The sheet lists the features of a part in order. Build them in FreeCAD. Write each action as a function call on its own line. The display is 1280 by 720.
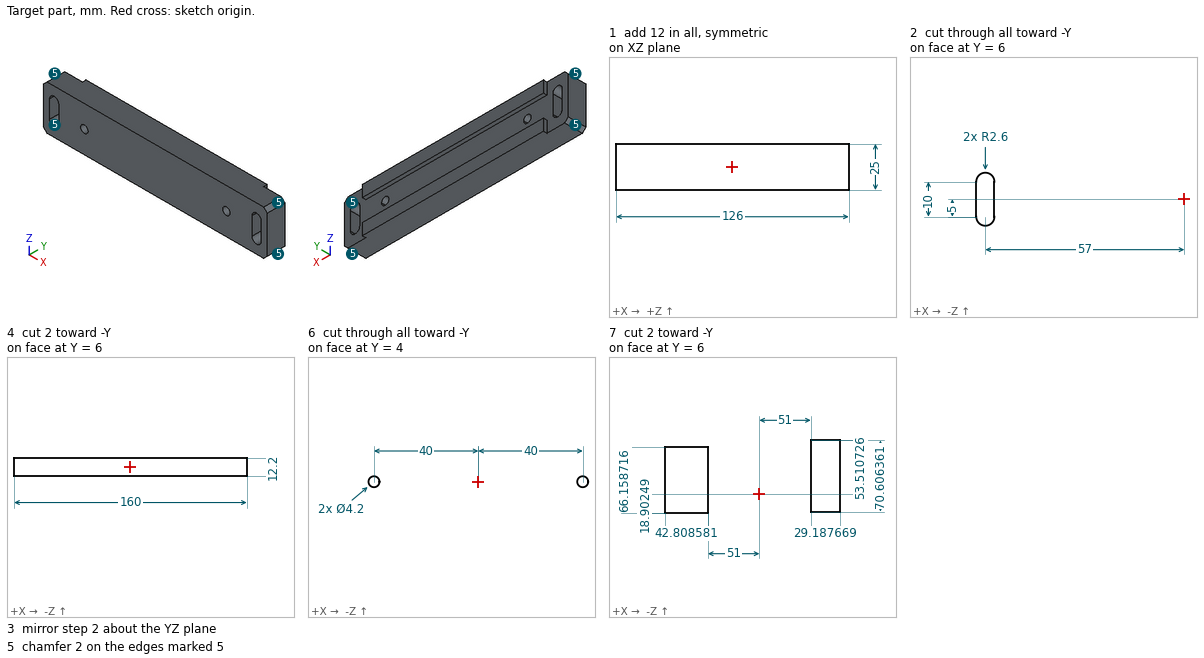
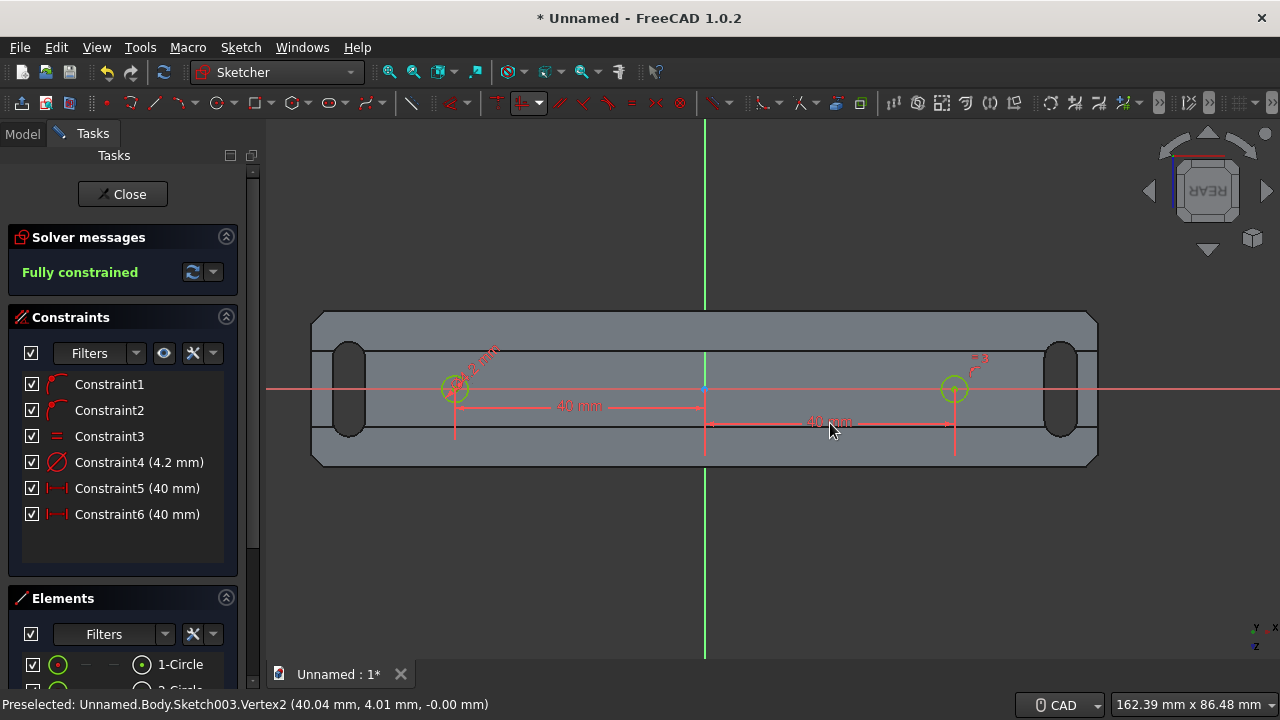
click(123, 194)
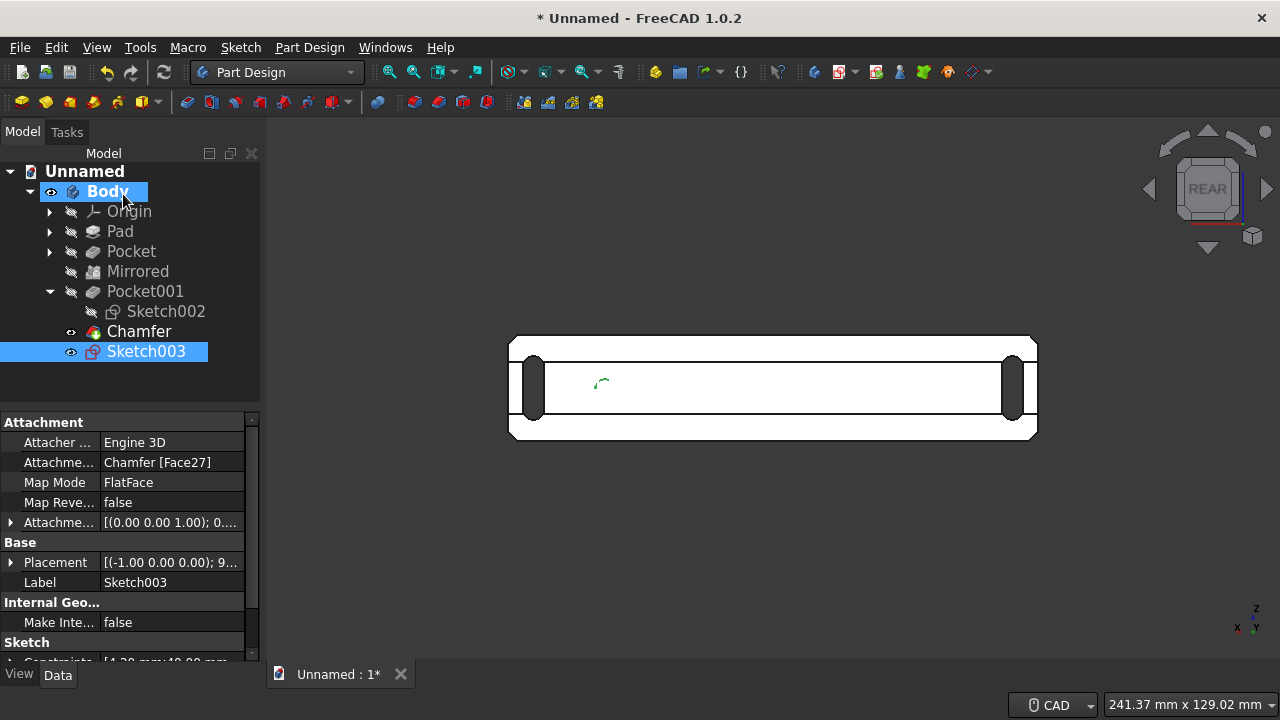
click(188, 102)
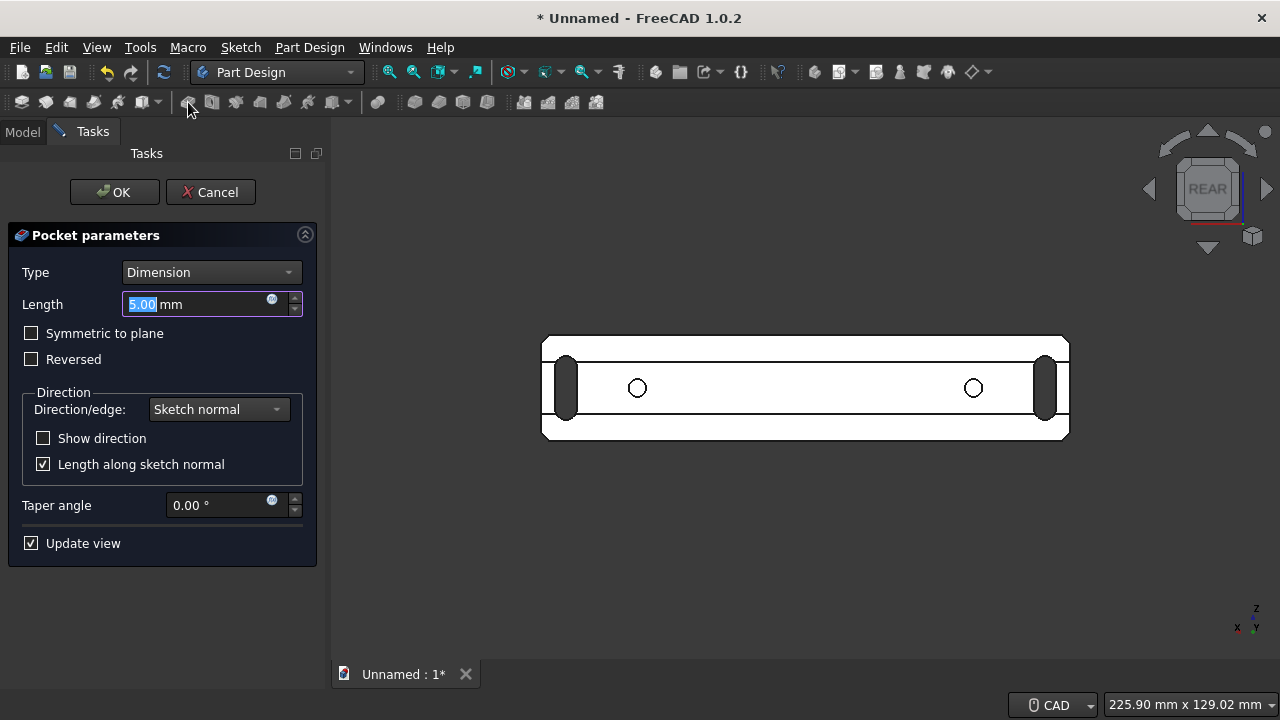
click(212, 272)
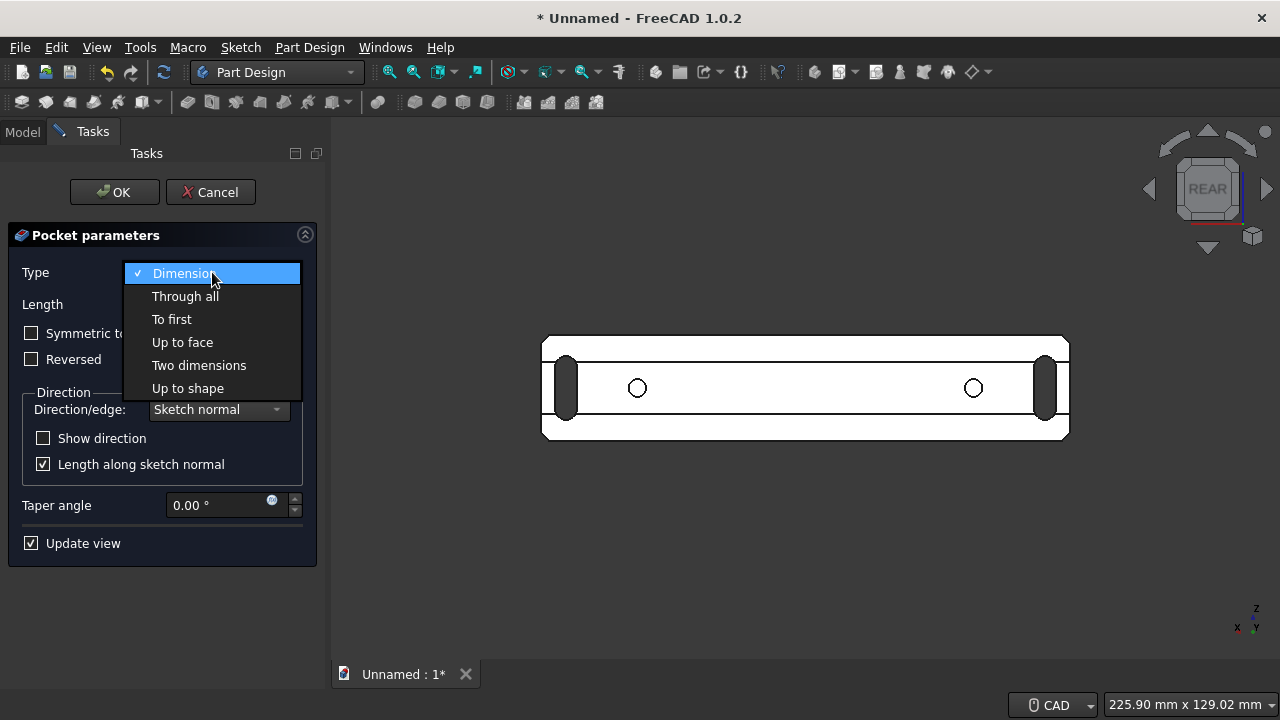
click(212, 296)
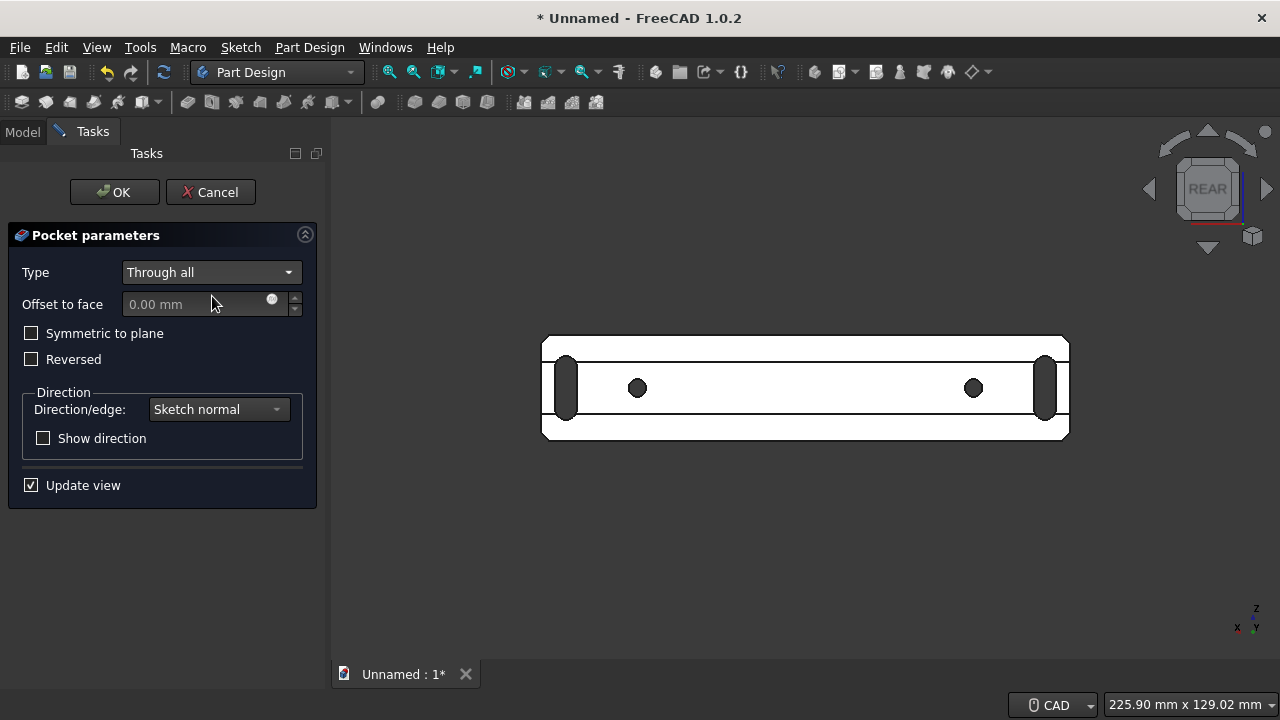
click(115, 192)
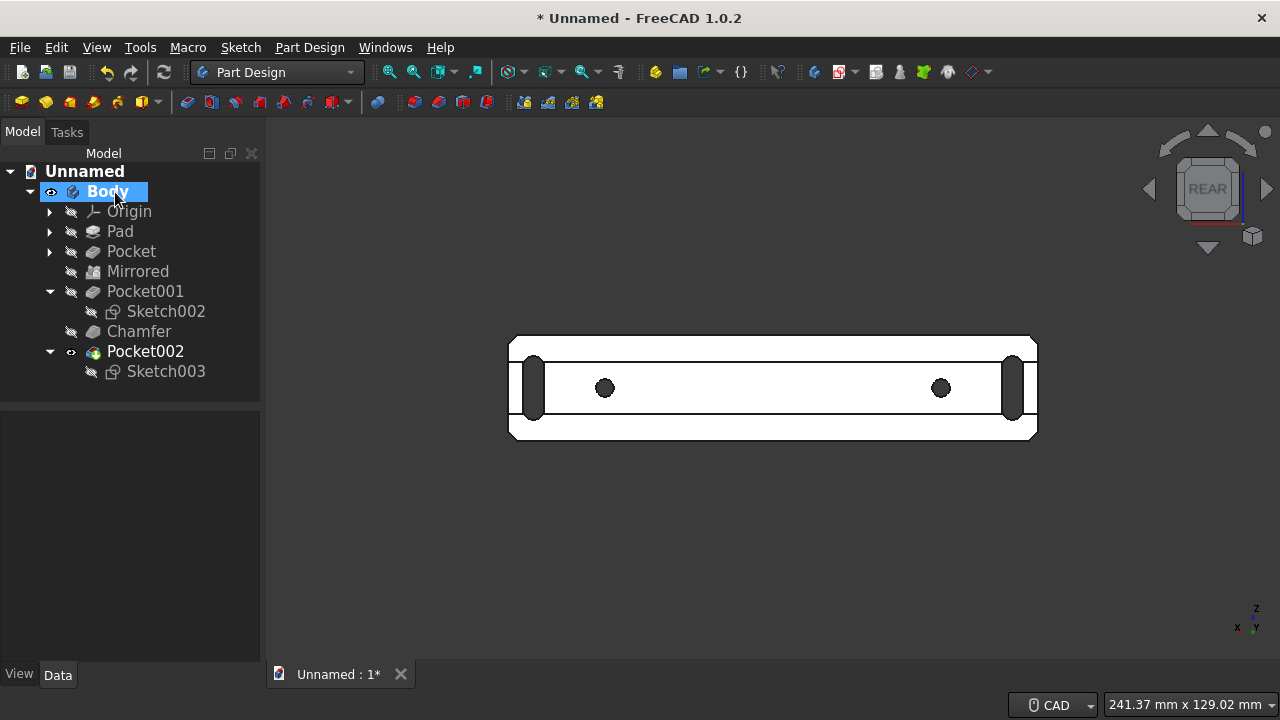
click(622, 426)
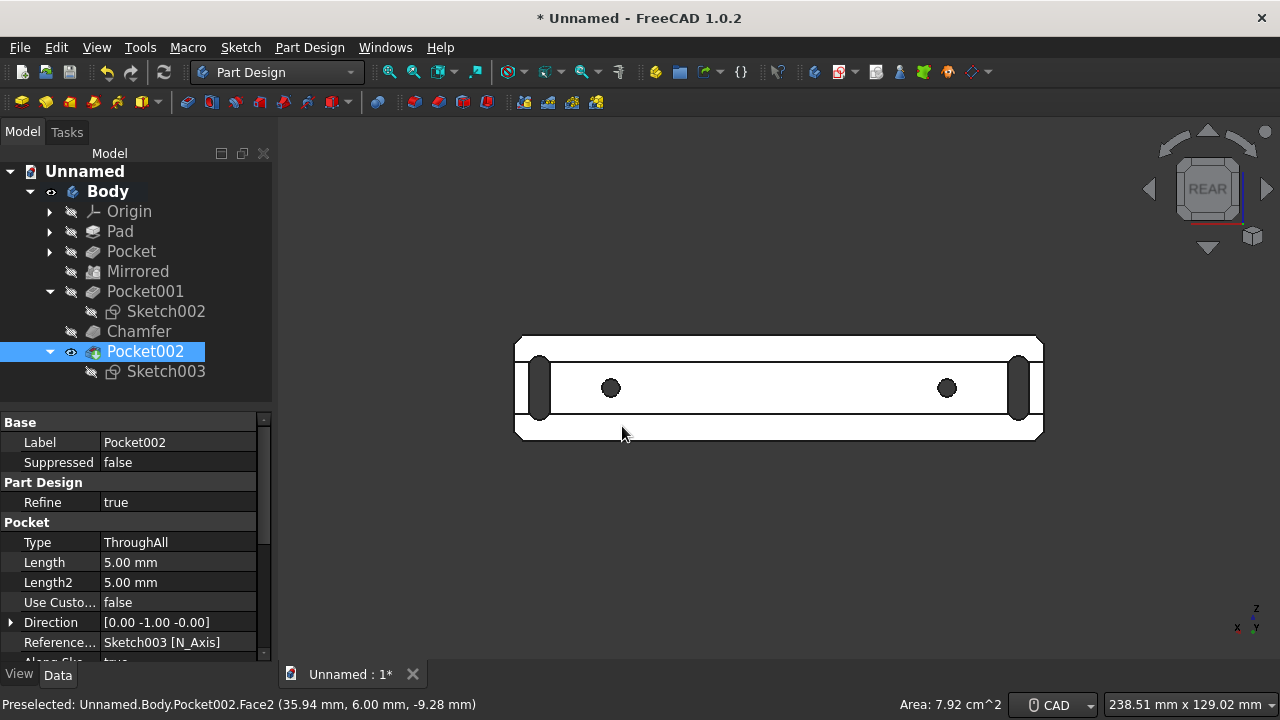
click(840, 72)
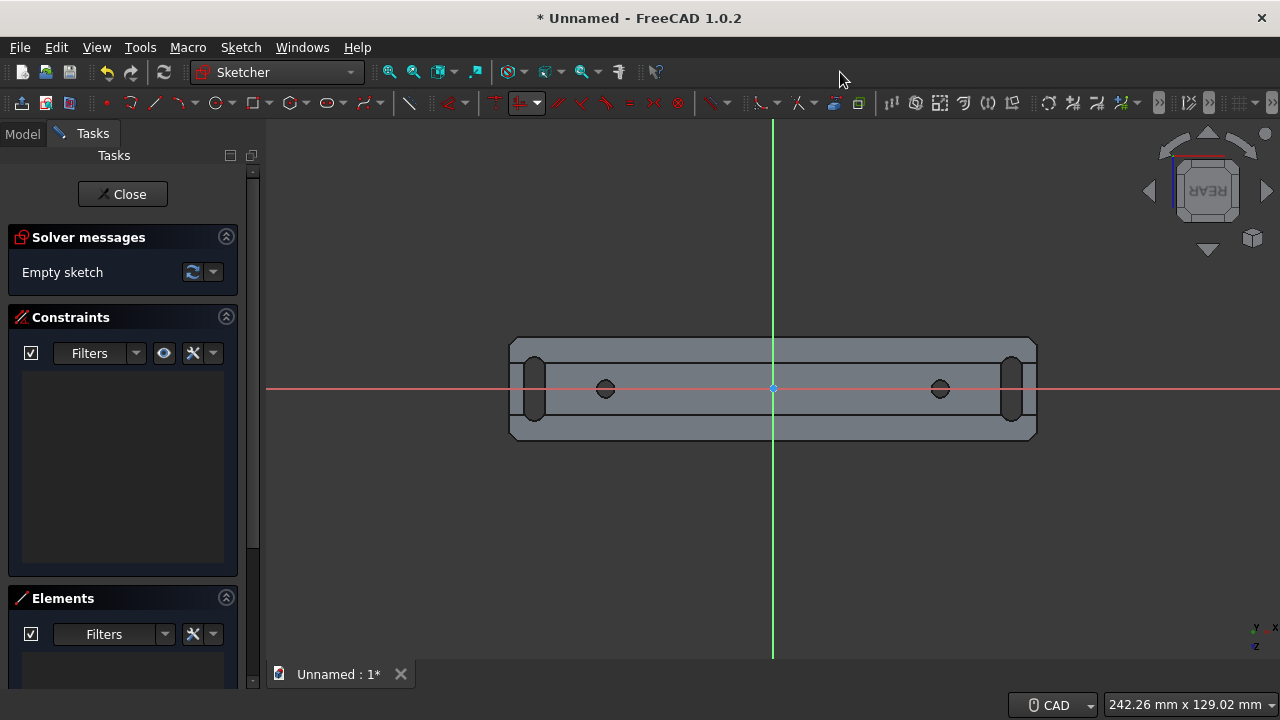
scroll(524, 631, down, 1)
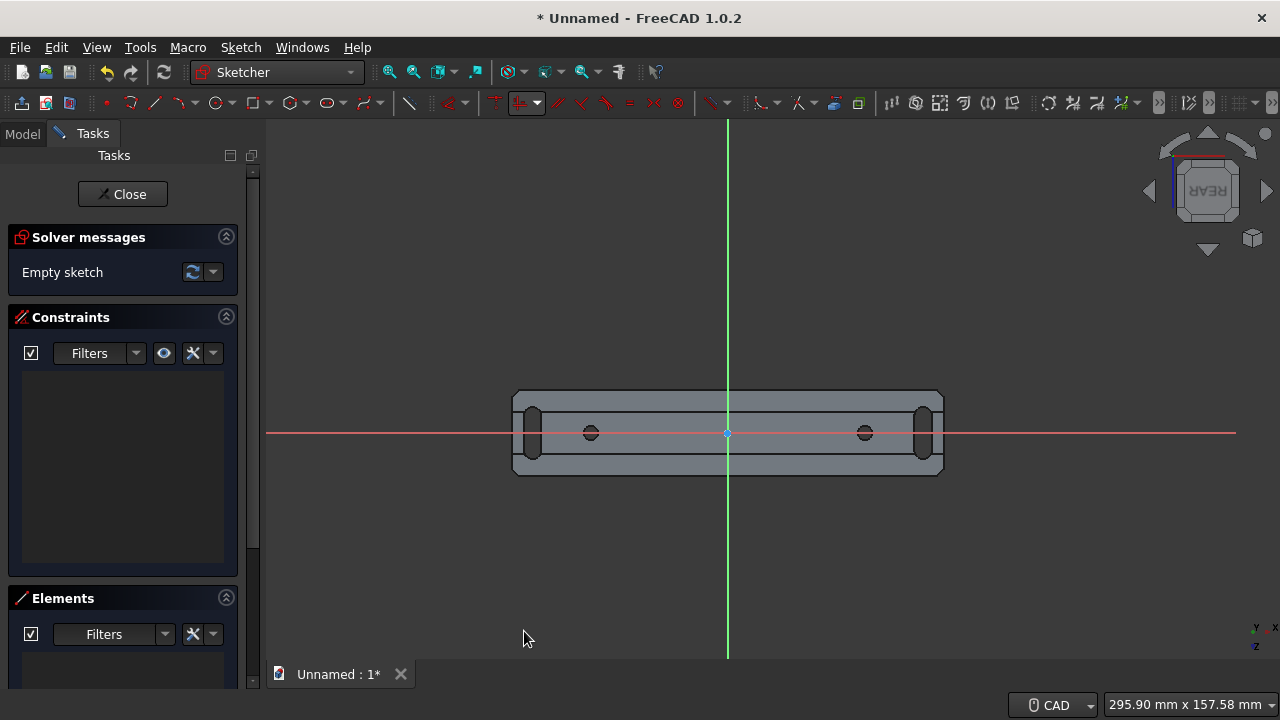
click(254, 104)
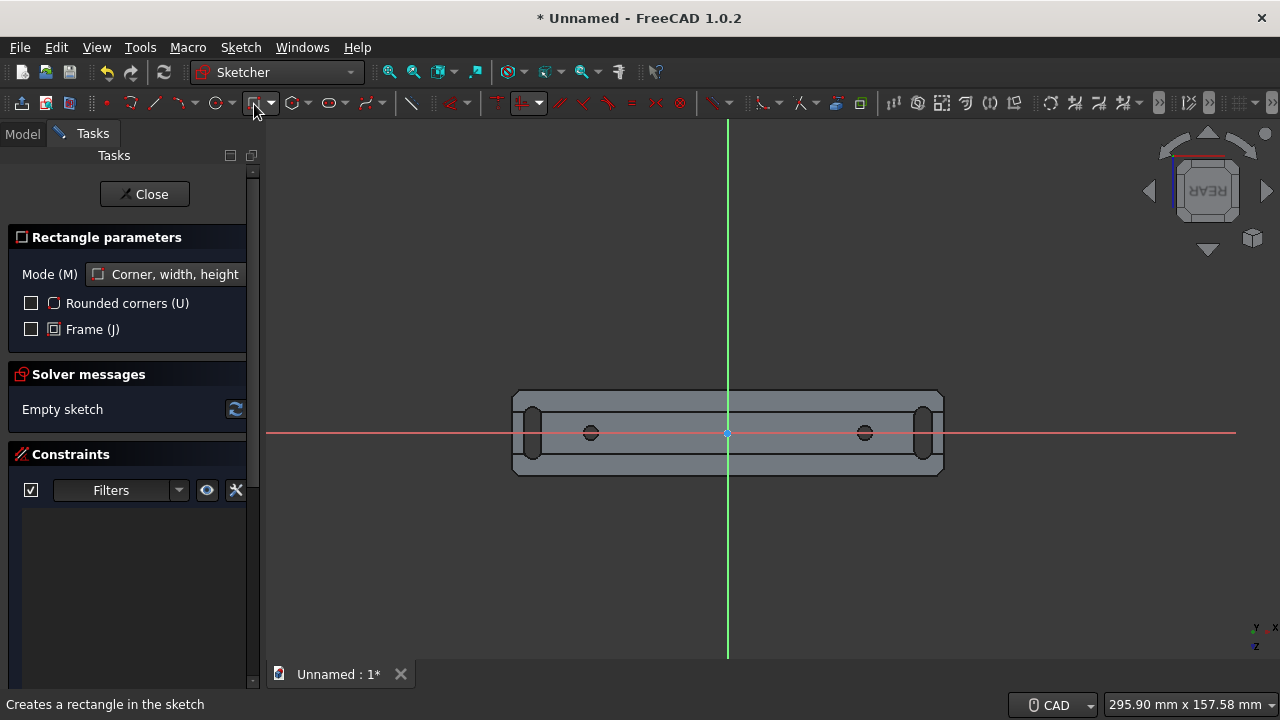
click(406, 271)
click(553, 498)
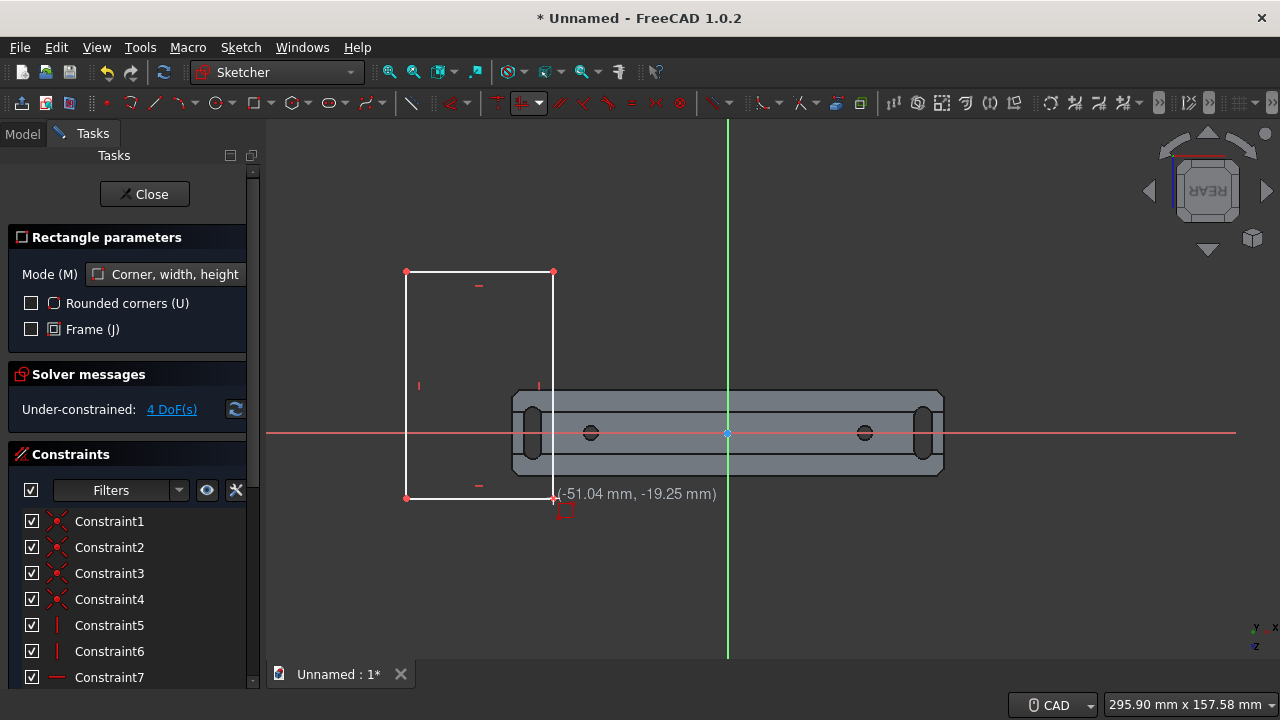
click(903, 250)
click(1003, 492)
key(Escape)